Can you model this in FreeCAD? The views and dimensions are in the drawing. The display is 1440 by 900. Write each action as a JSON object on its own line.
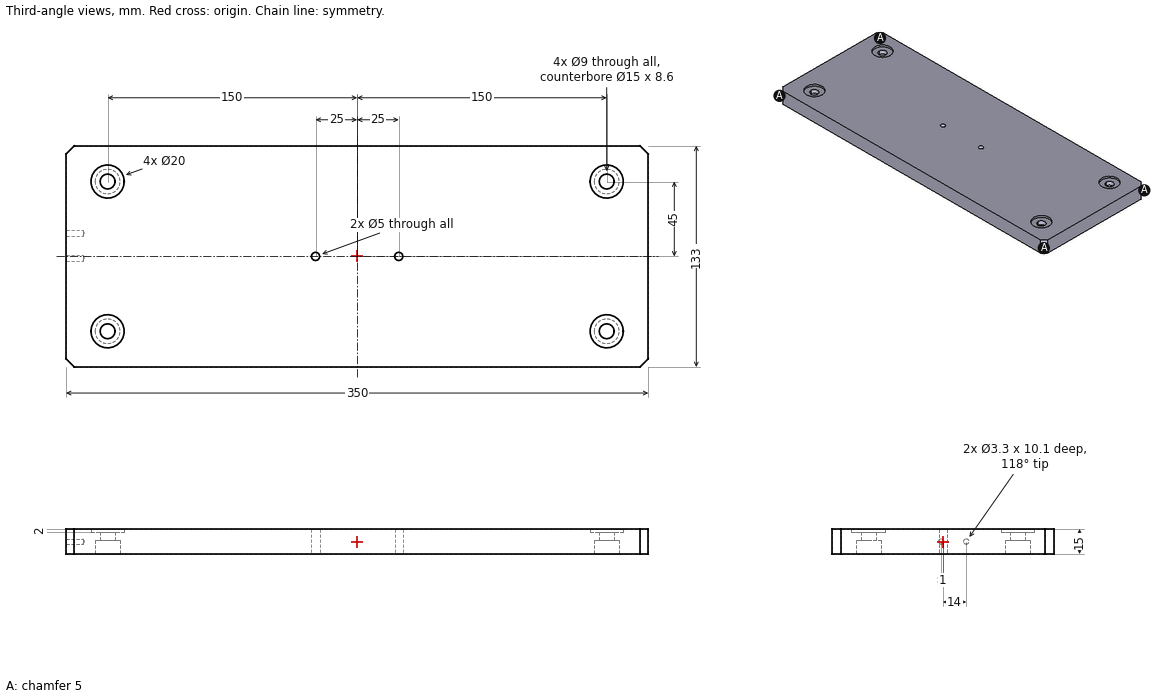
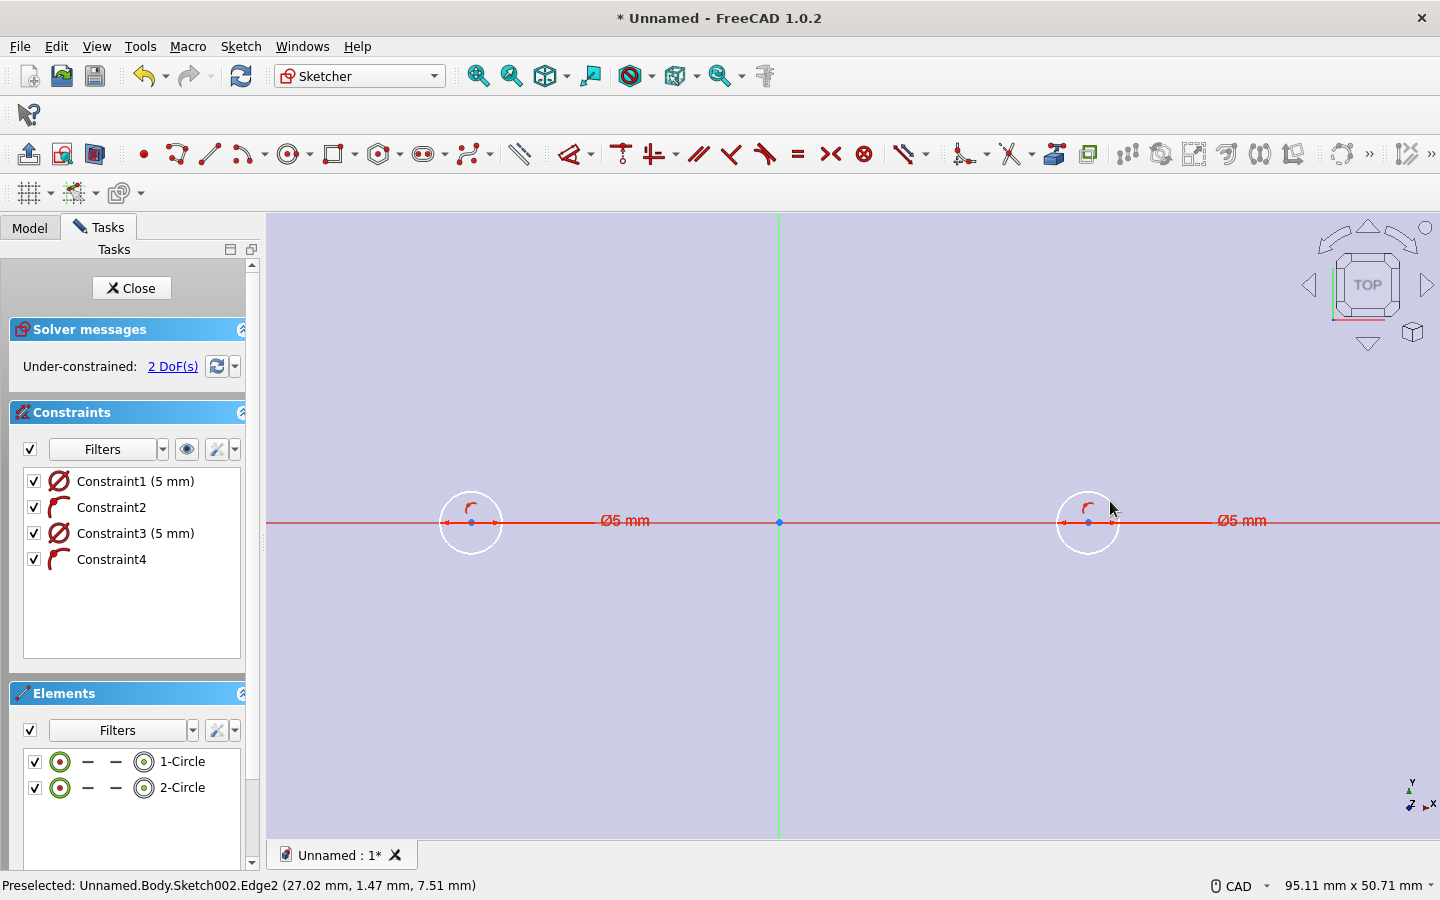
{"action": "key", "text": "d"}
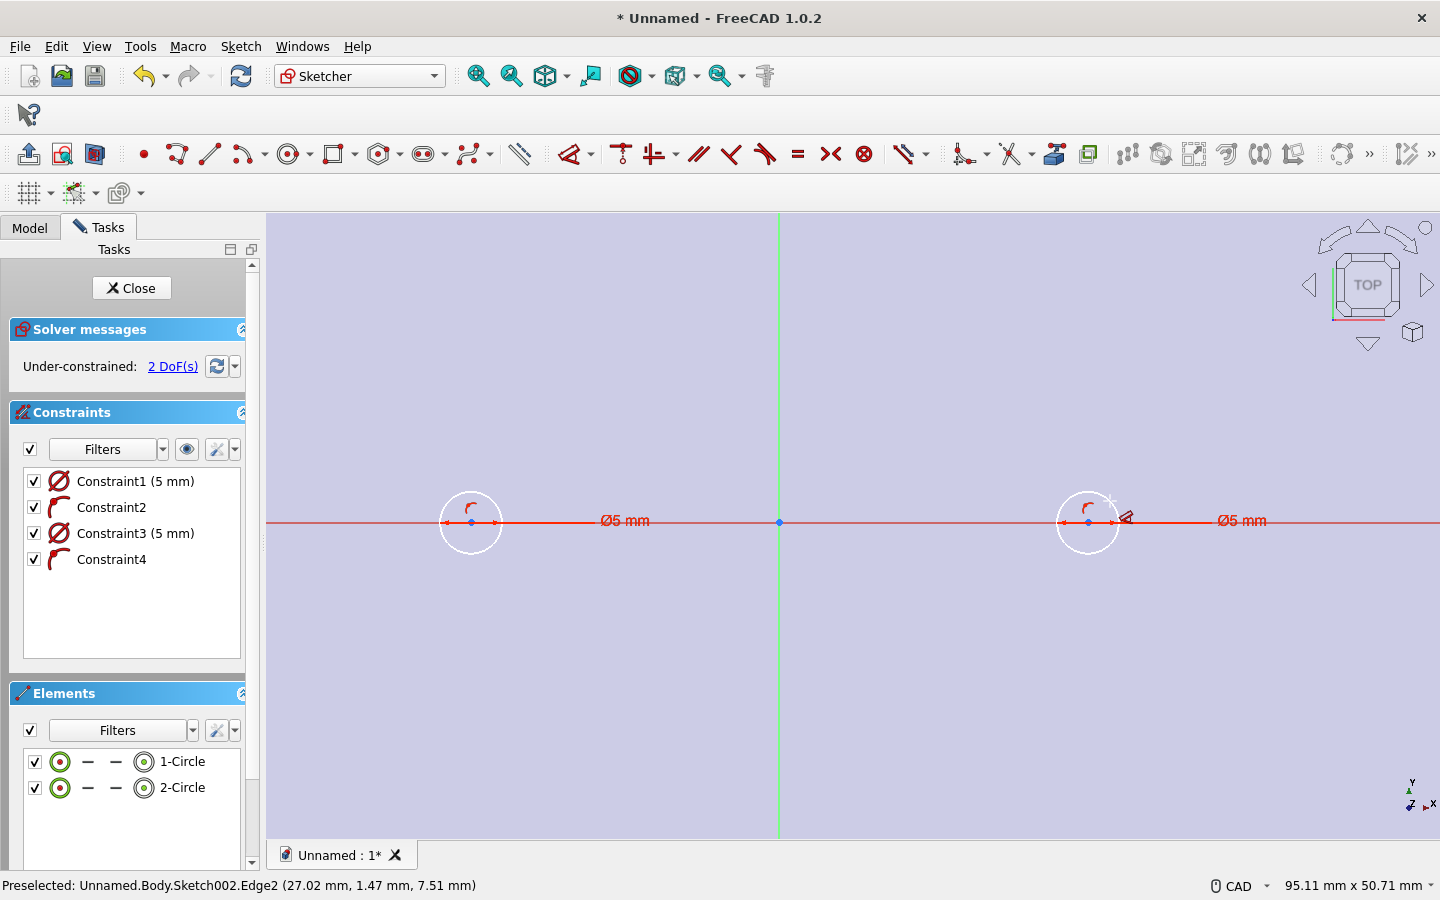
{"action": "left_click", "coordinate": [471, 523]}
{"action": "left_click", "coordinate": [625, 557]}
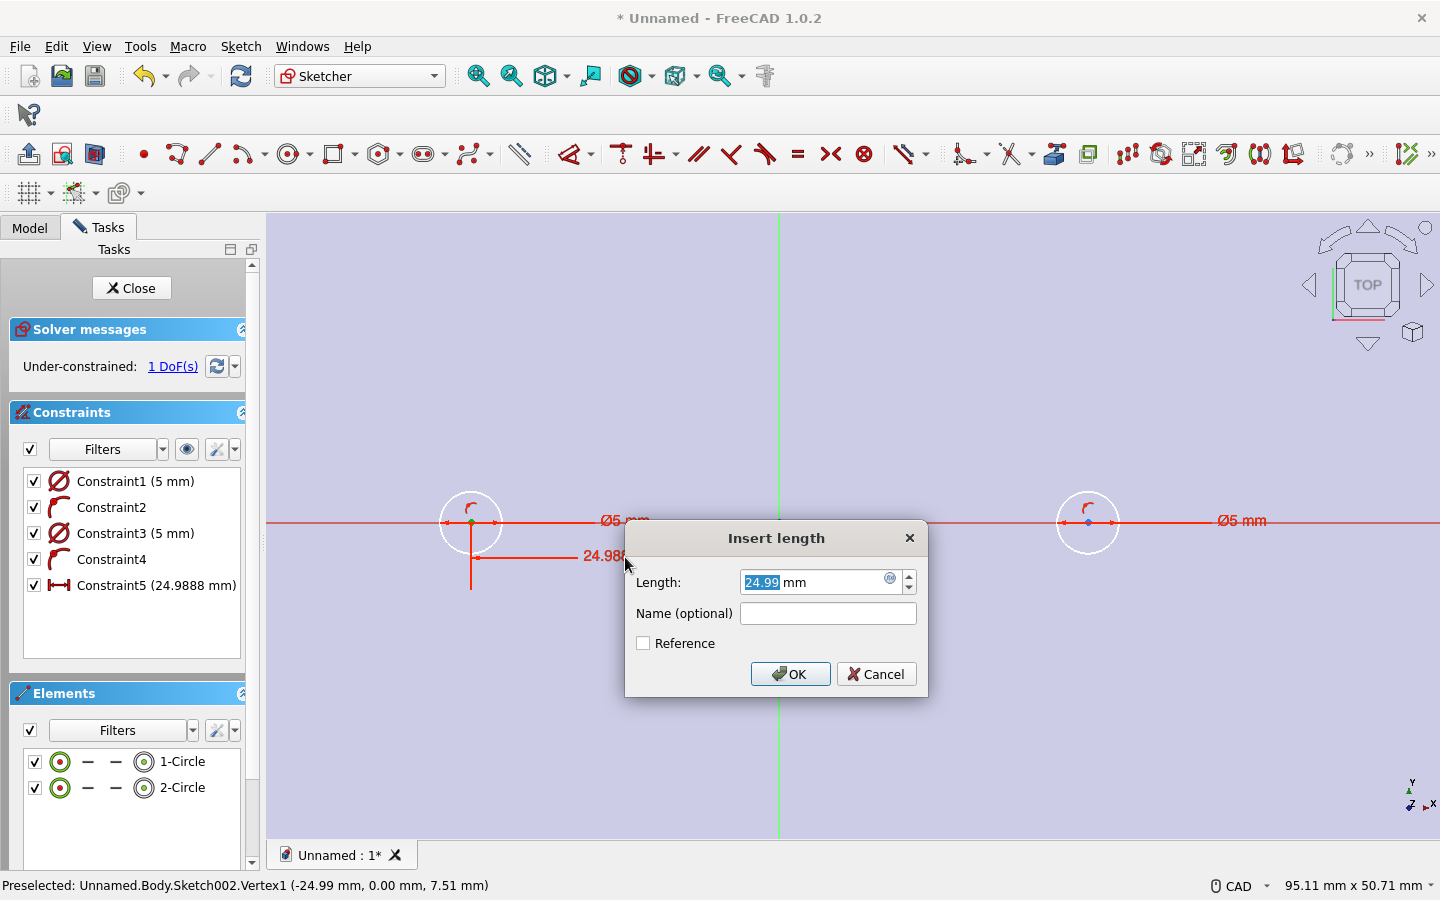
{"action": "type", "text": "25"}
{"action": "key", "text": "Return"}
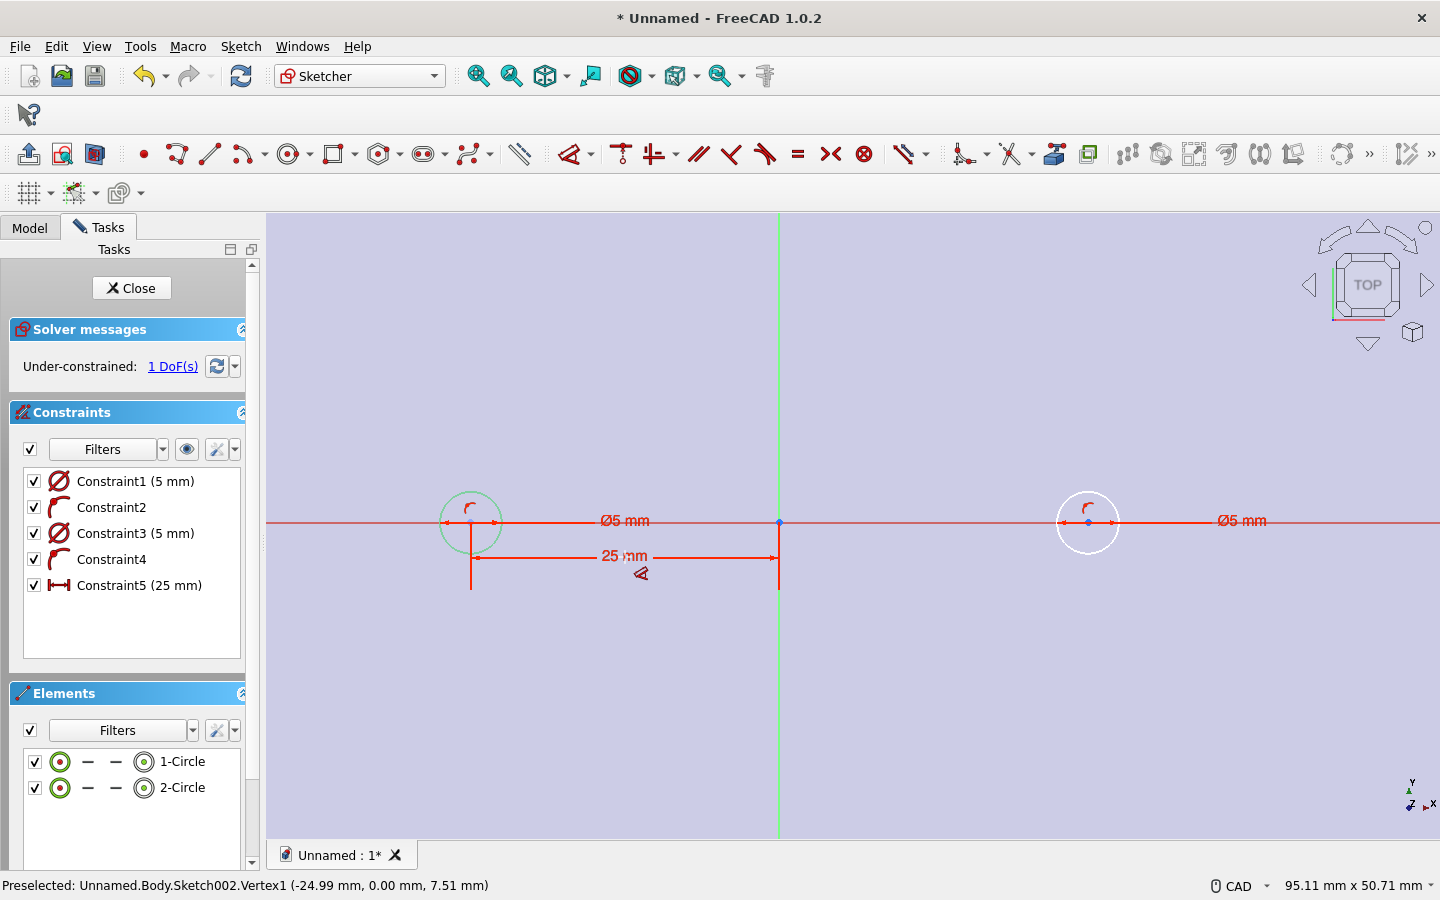
{"action": "left_click", "coordinate": [1088, 523]}
{"action": "left_click", "coordinate": [934, 557]}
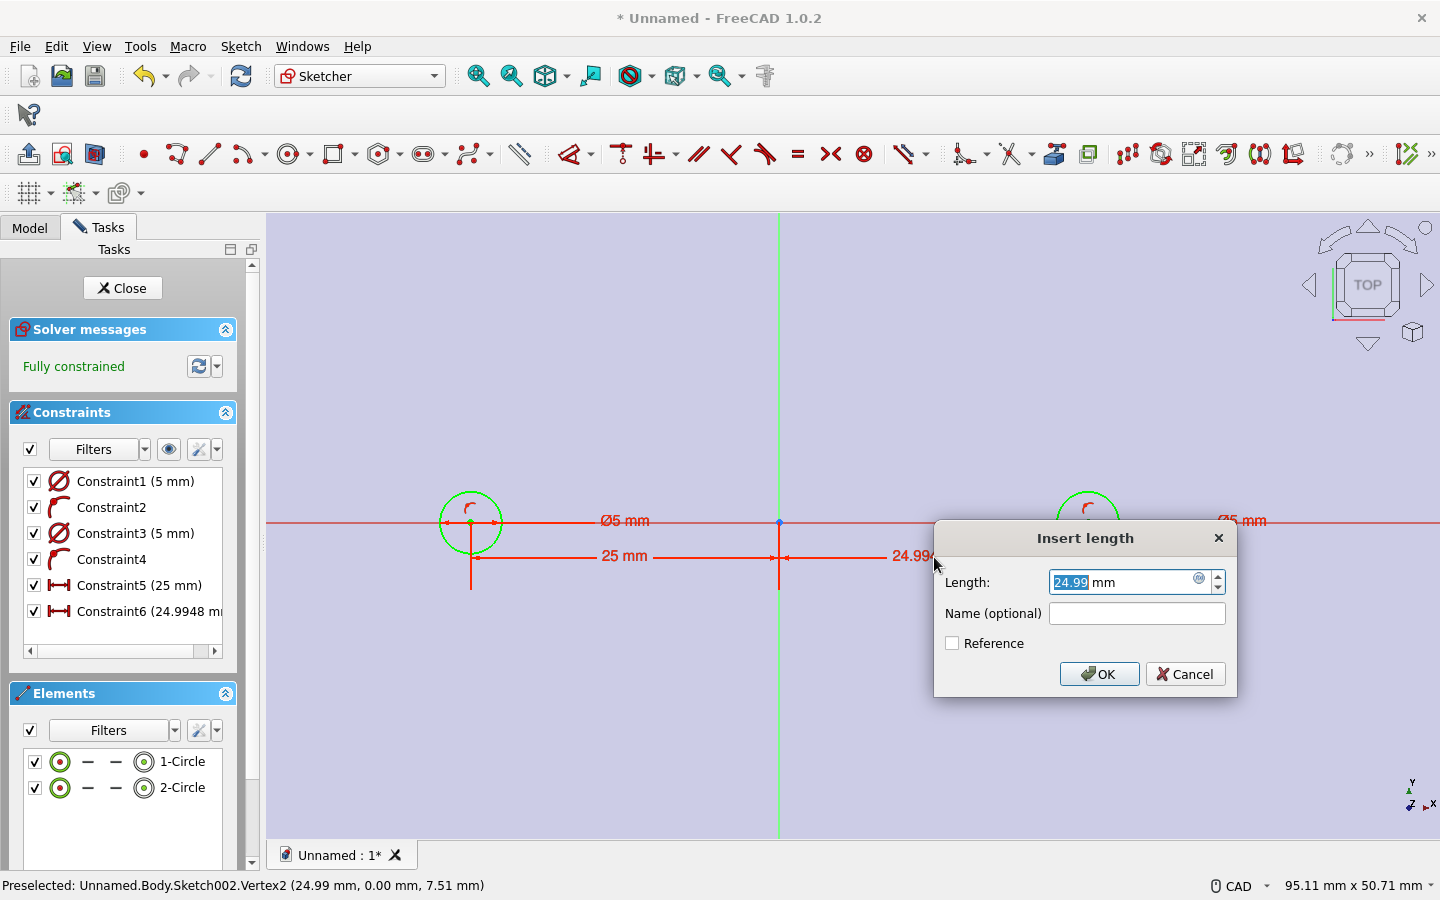
{"action": "type", "text": "25"}
{"action": "key", "text": "Return"}
{"action": "key", "text": "Escape"}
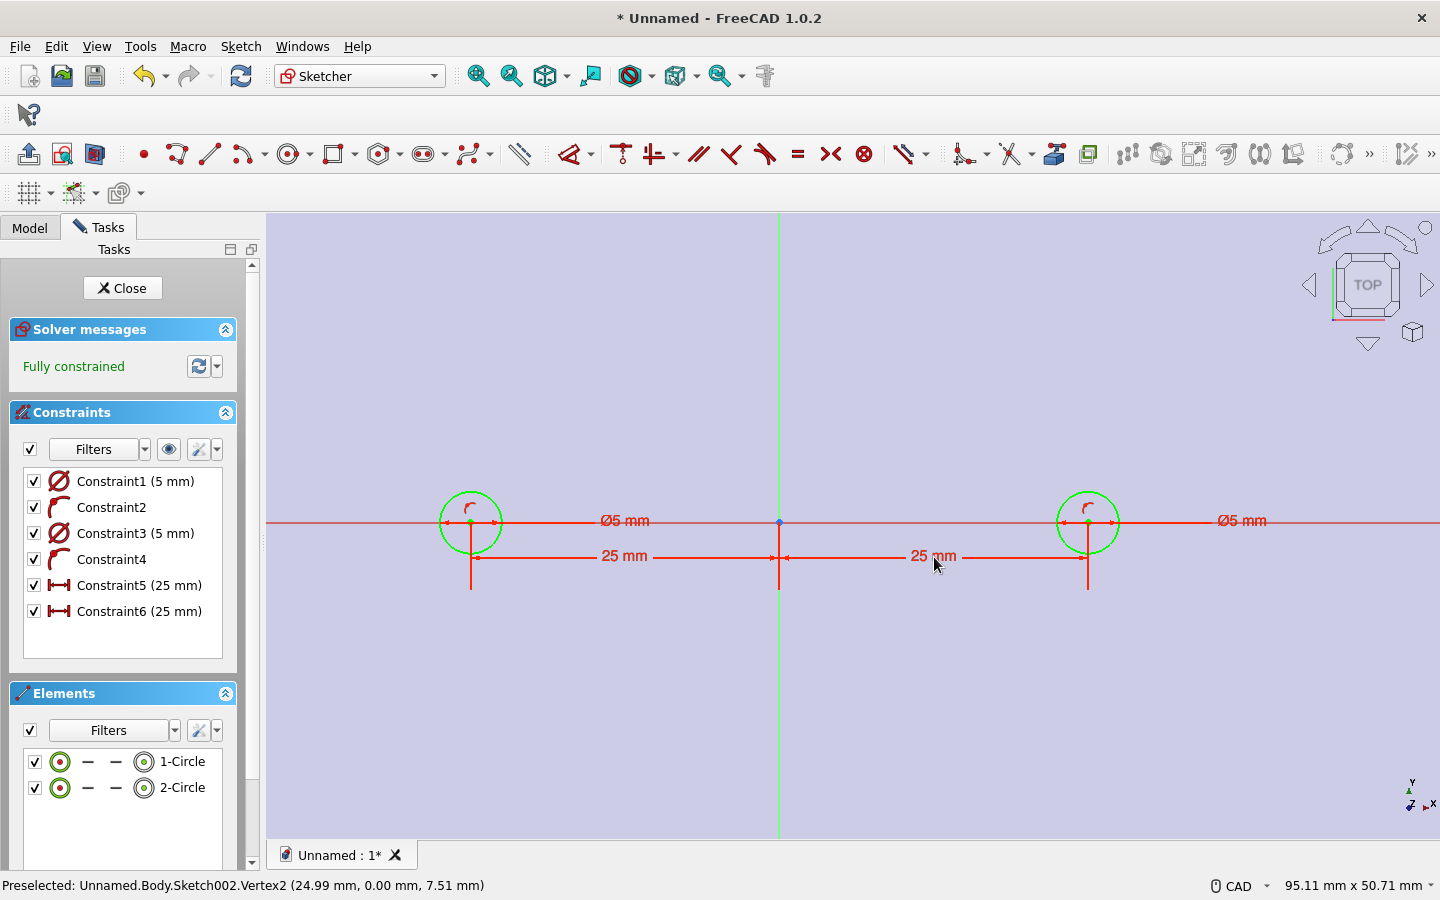
{"action": "left_click", "coordinate": [123, 288]}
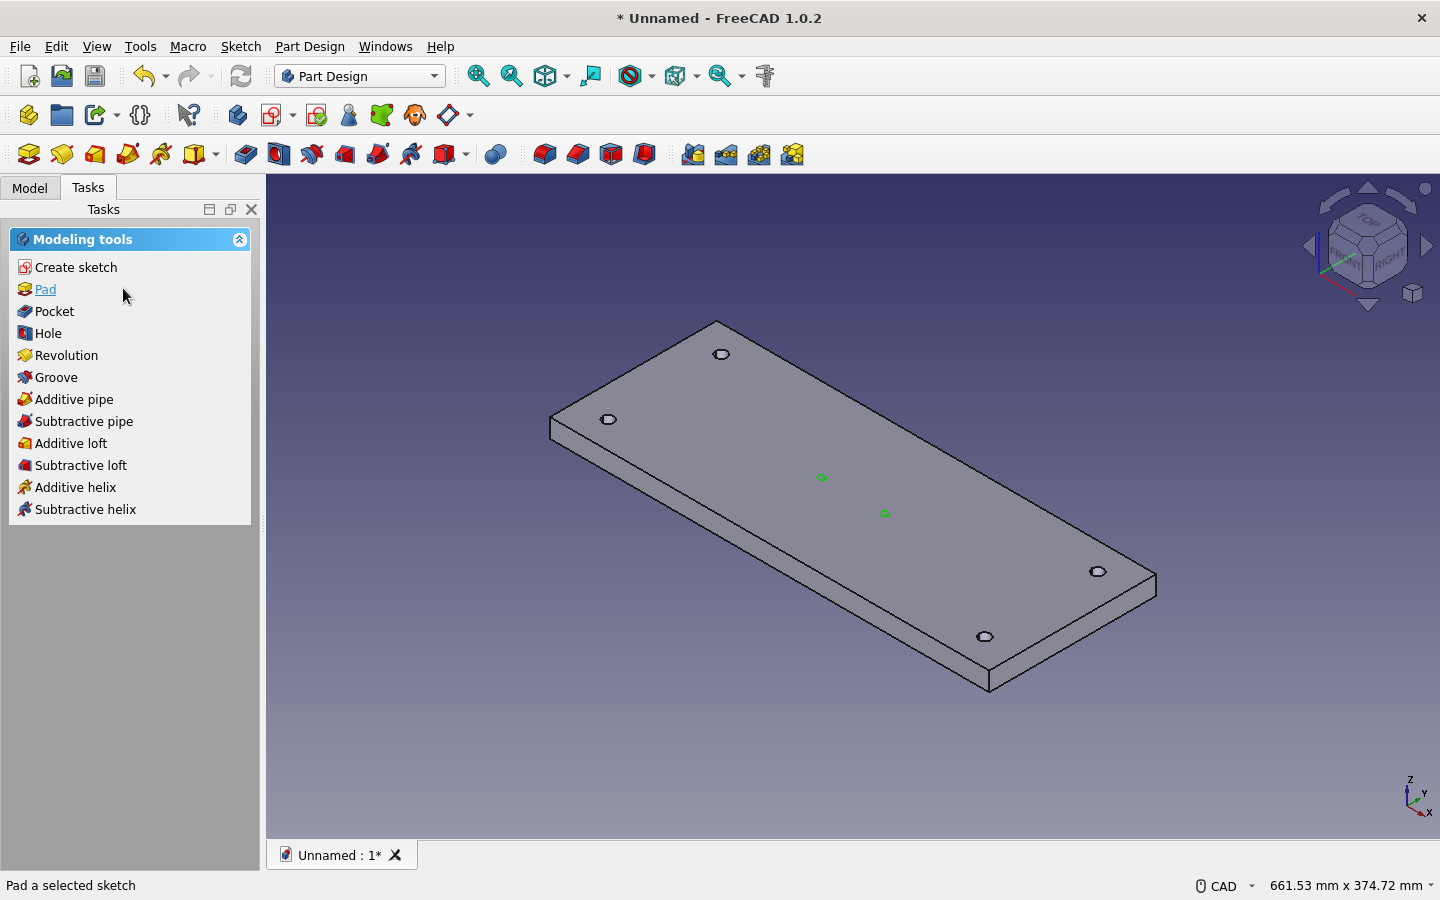
{"action": "left_click", "coordinate": [279, 154]}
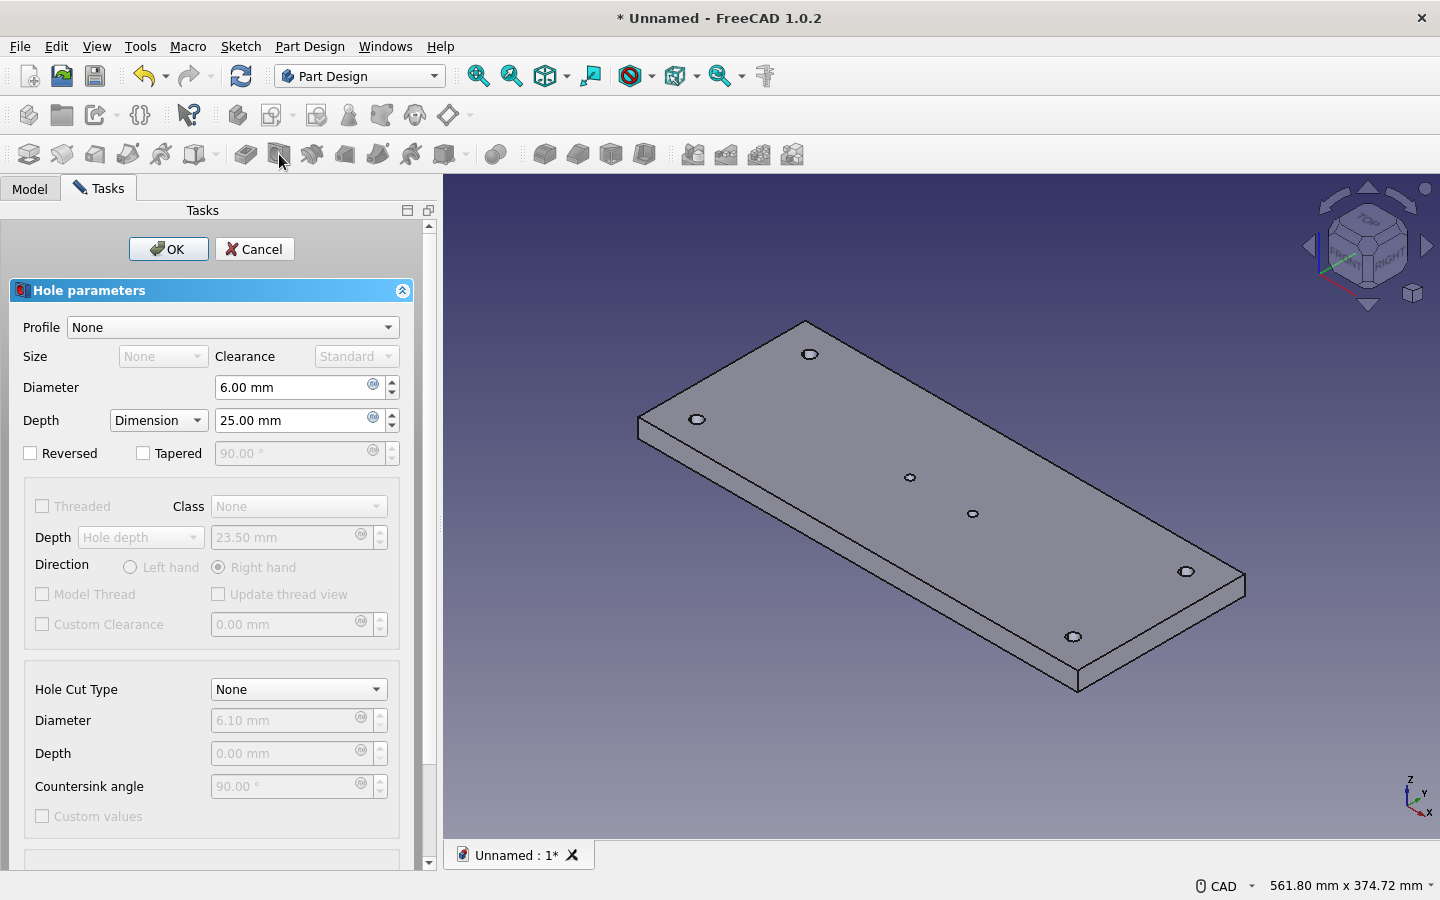
{"action": "triple_click", "coordinate": [300, 388]}